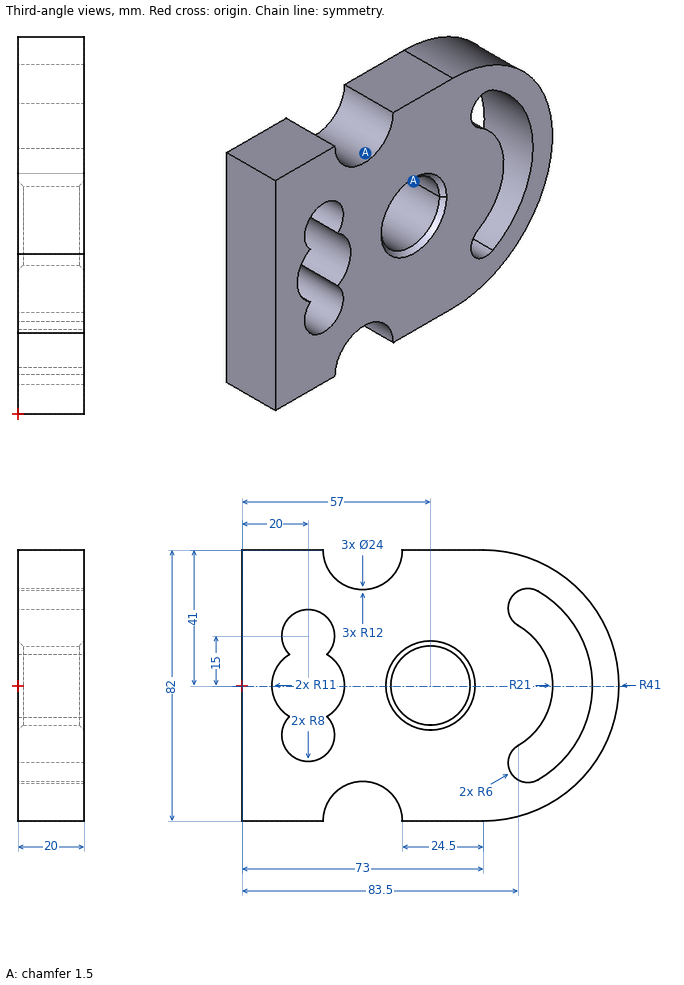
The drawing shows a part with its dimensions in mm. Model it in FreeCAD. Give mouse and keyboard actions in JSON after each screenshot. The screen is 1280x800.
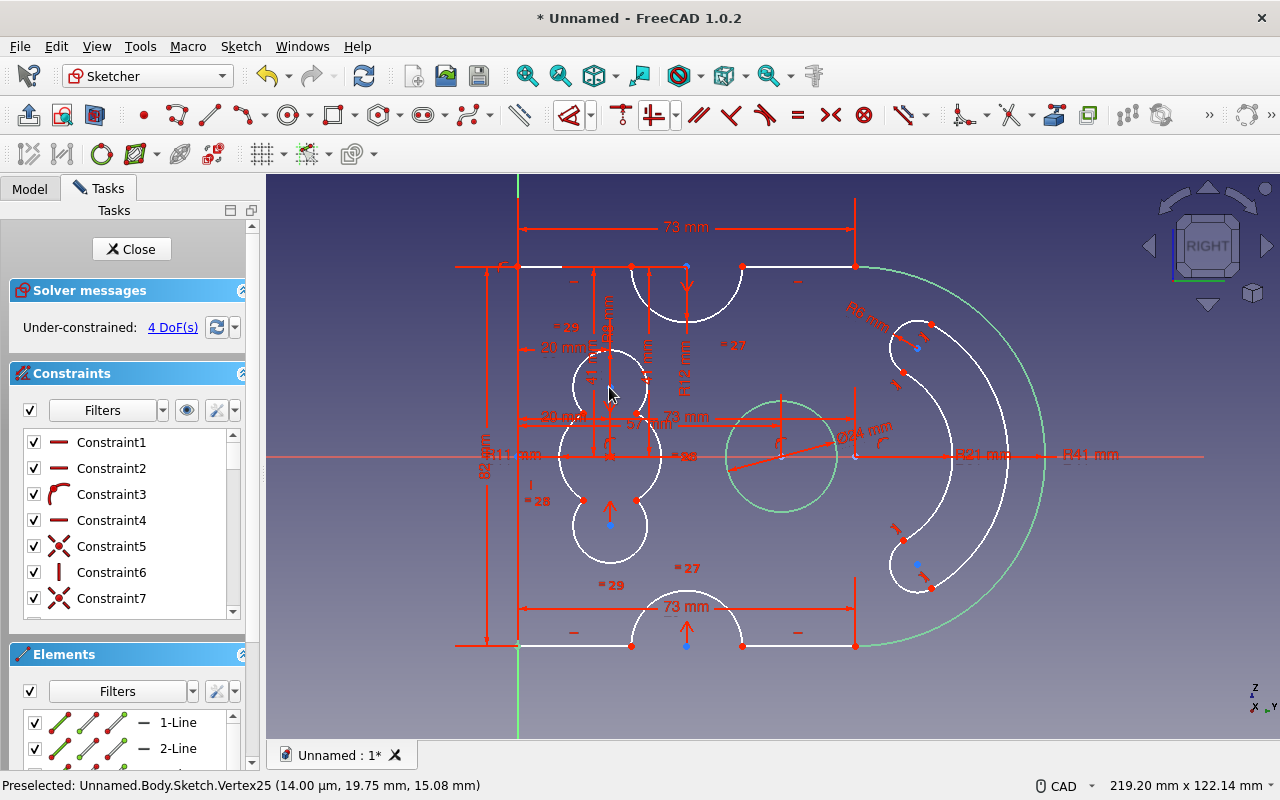
{"action": "left_click", "coordinate": [610, 387]}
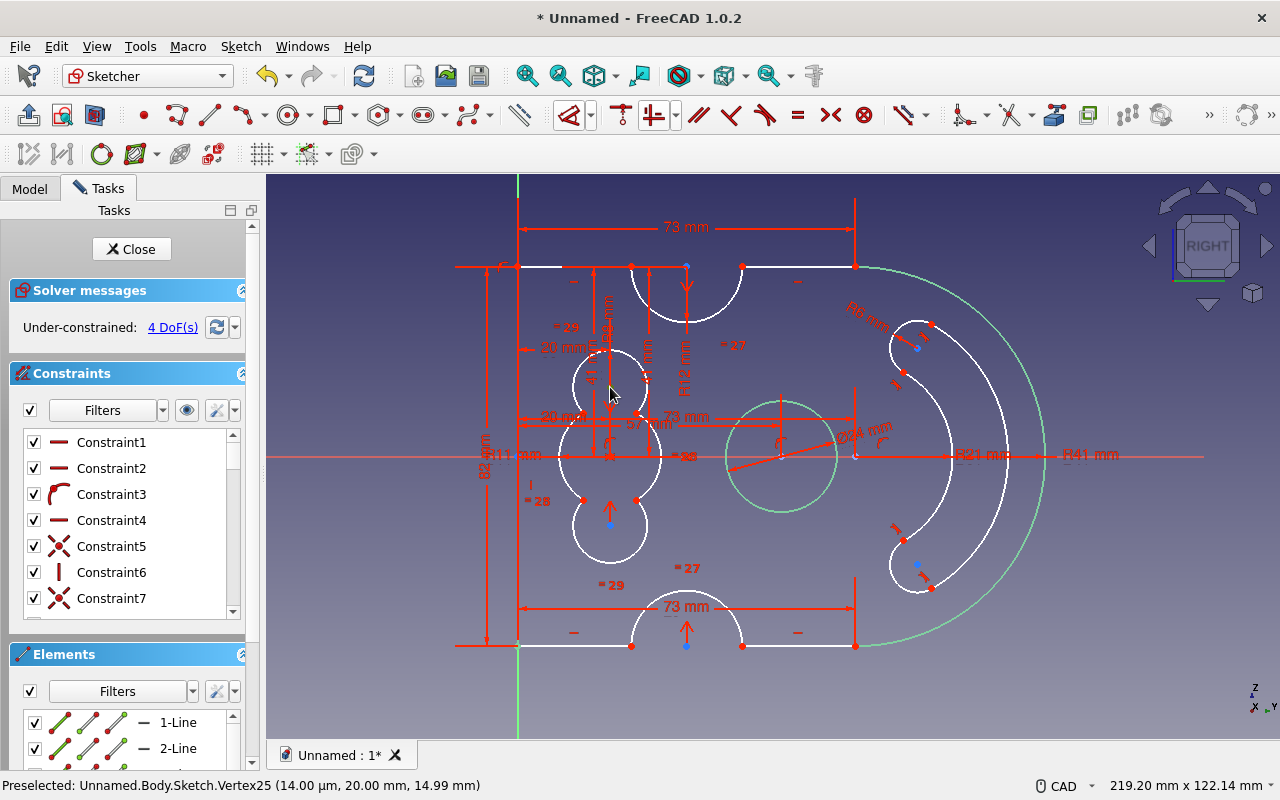
{"action": "key", "text": "i"}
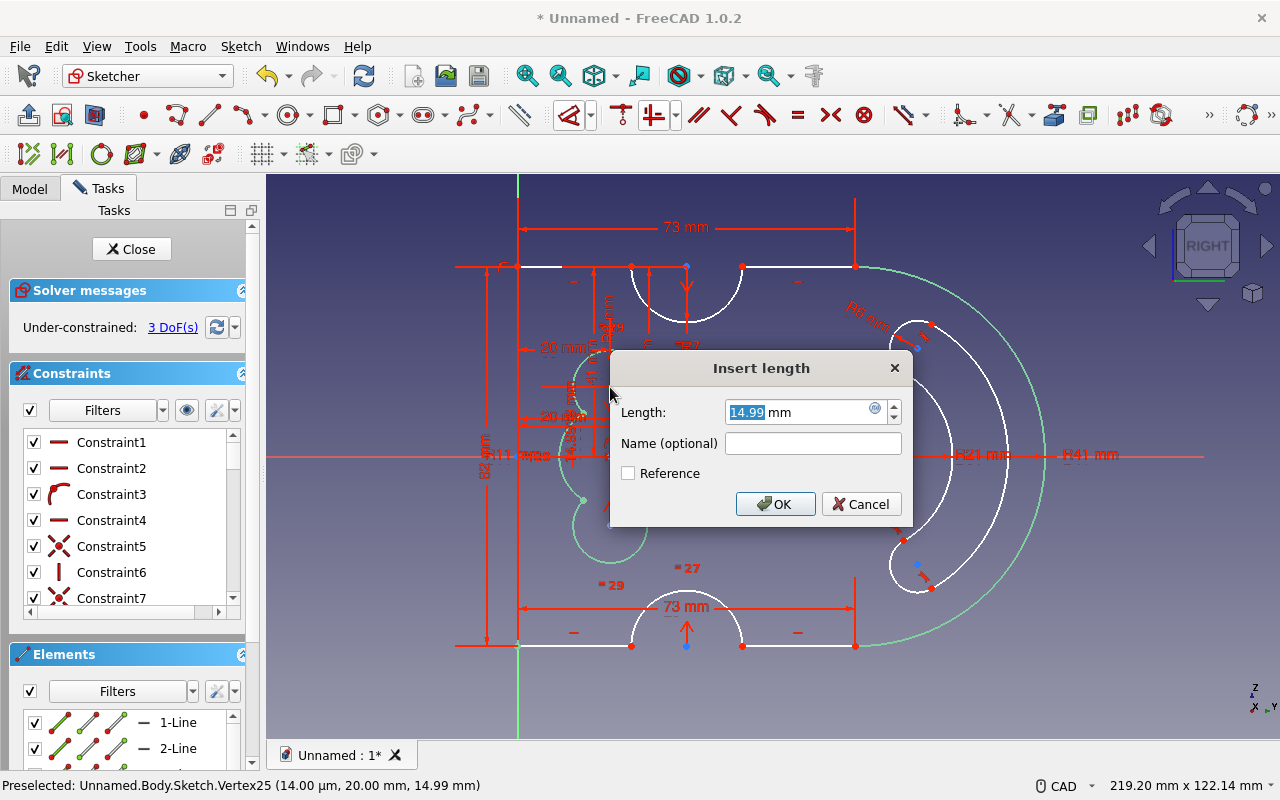
{"action": "type", "text": "15"}
{"action": "key", "text": "Return"}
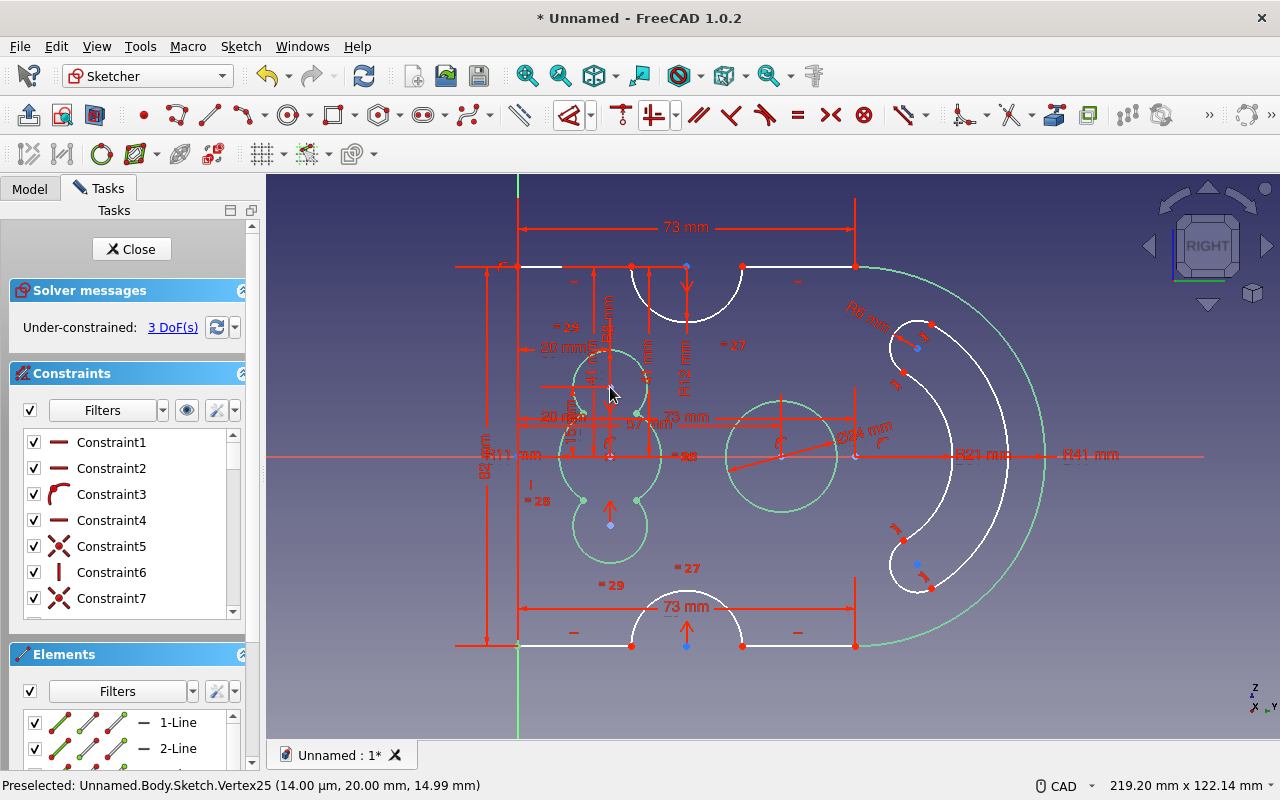
{"action": "left_click", "coordinate": [776, 646]}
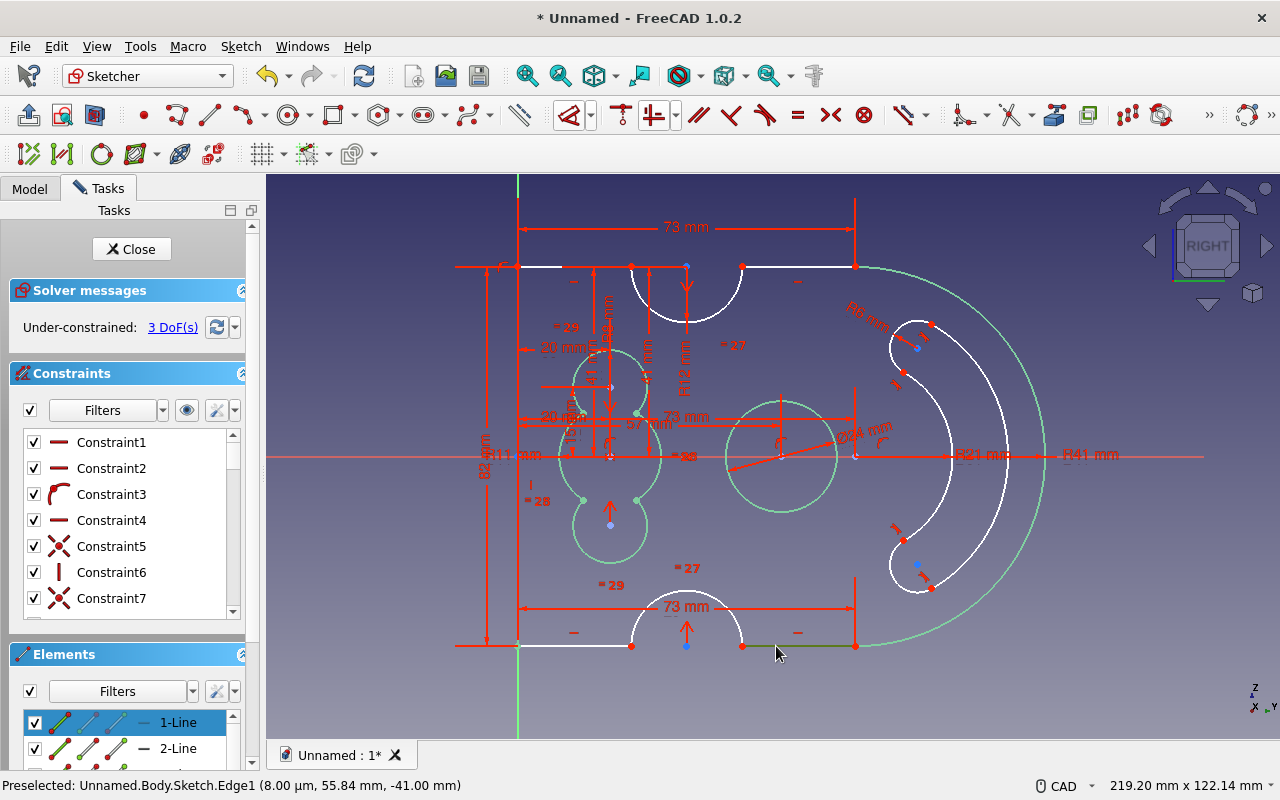
{"action": "key", "text": "l"}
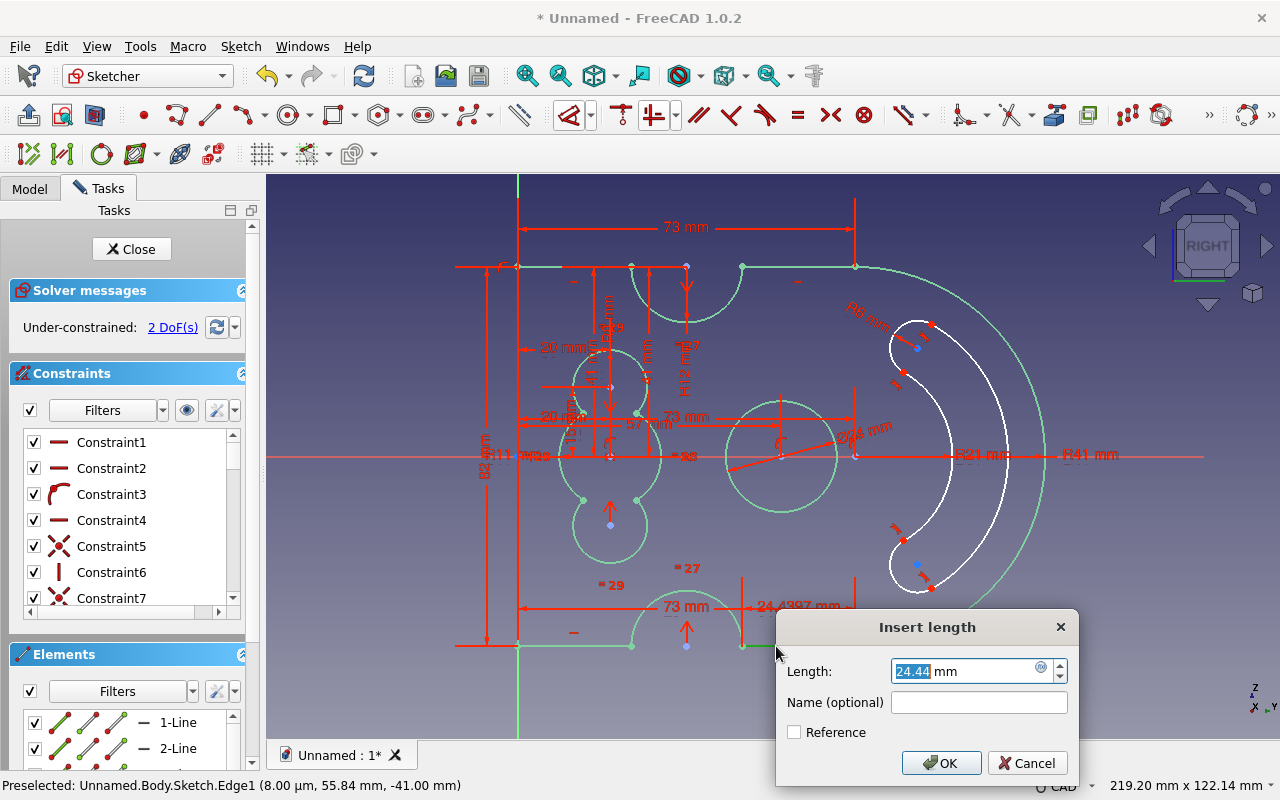
{"action": "type", "text": "24.5"}
{"action": "key", "text": "Return"}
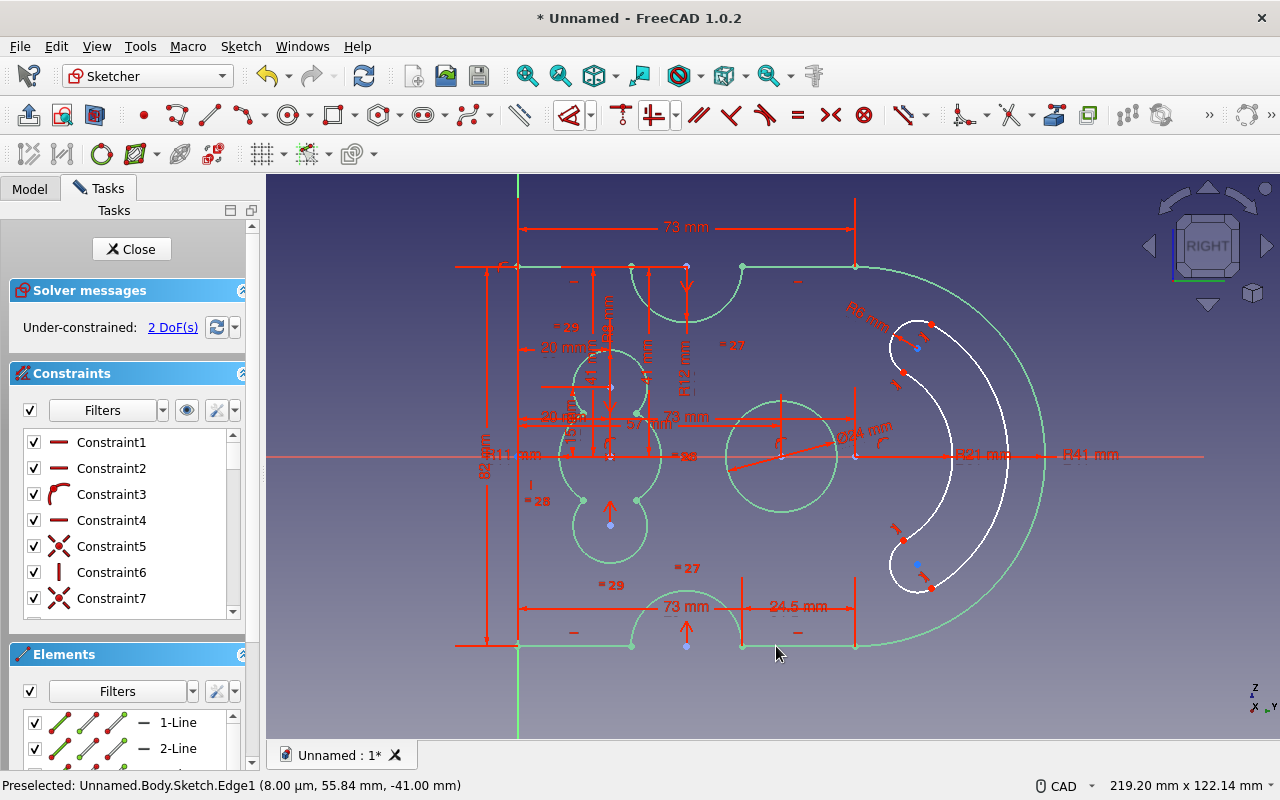
{"action": "left_click", "coordinate": [904, 541]}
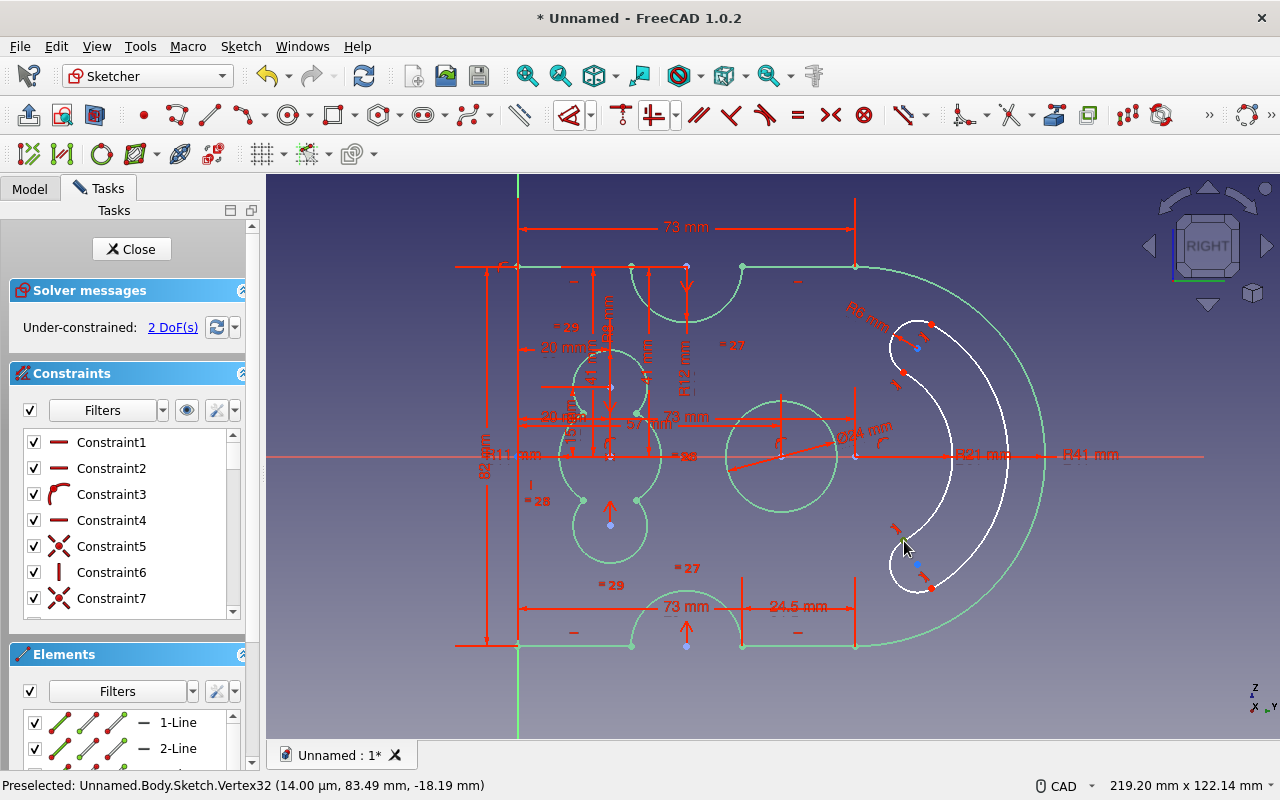
{"action": "key", "text": "l"}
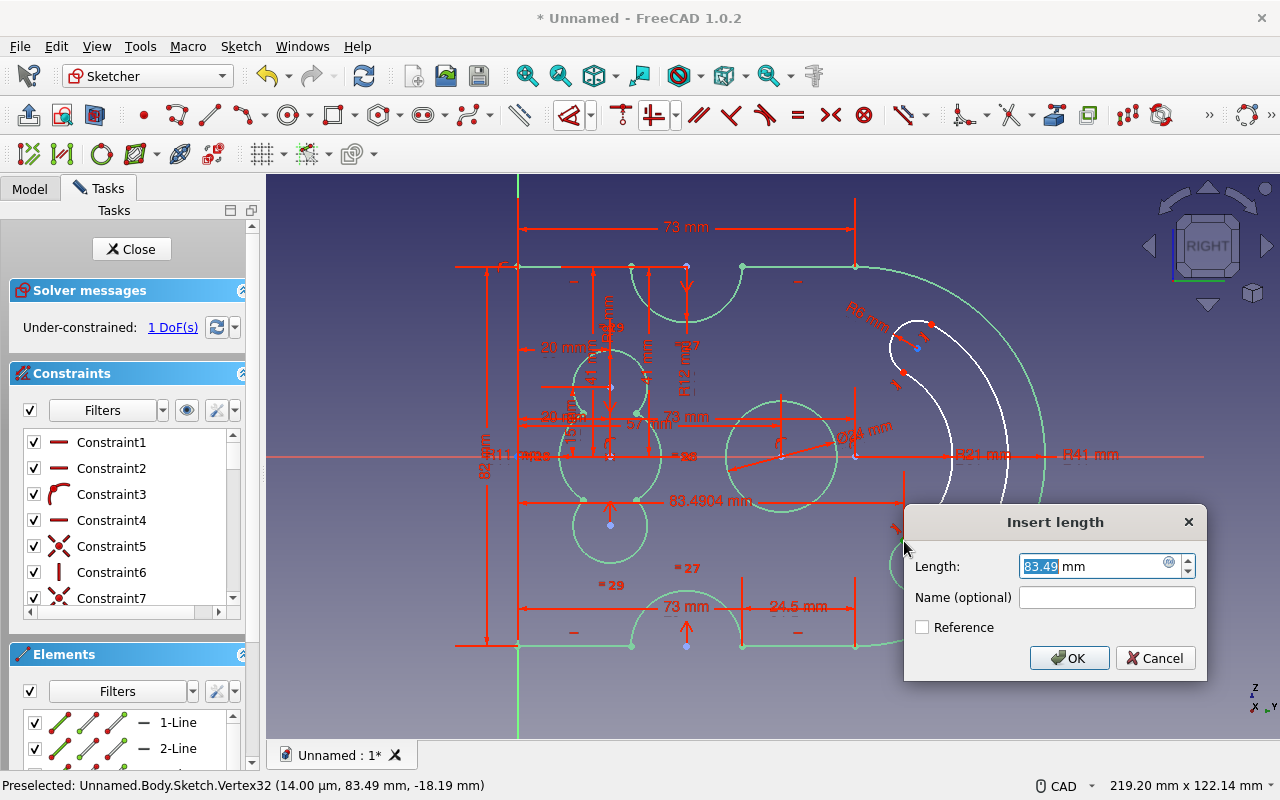
{"action": "type", "text": "83.5"}
{"action": "key", "text": "Return"}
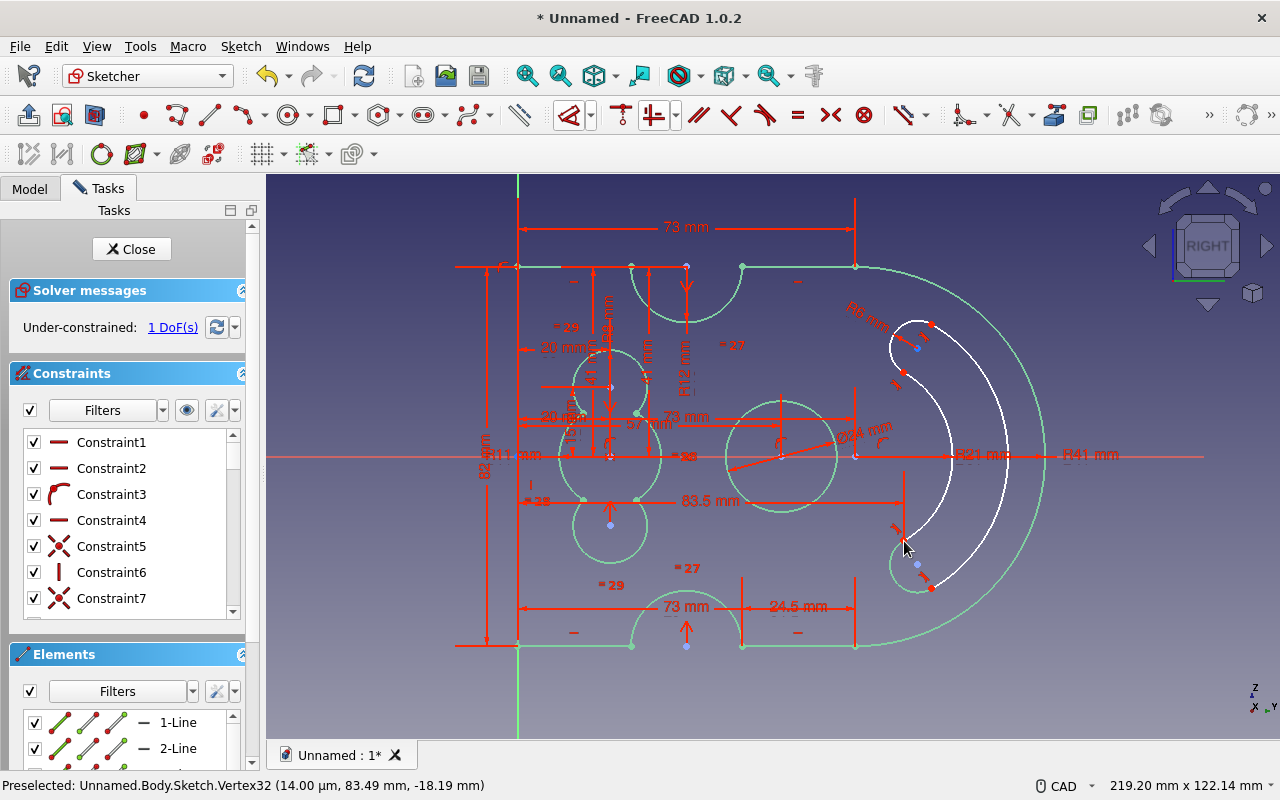
{"action": "left_click", "coordinate": [904, 372]}